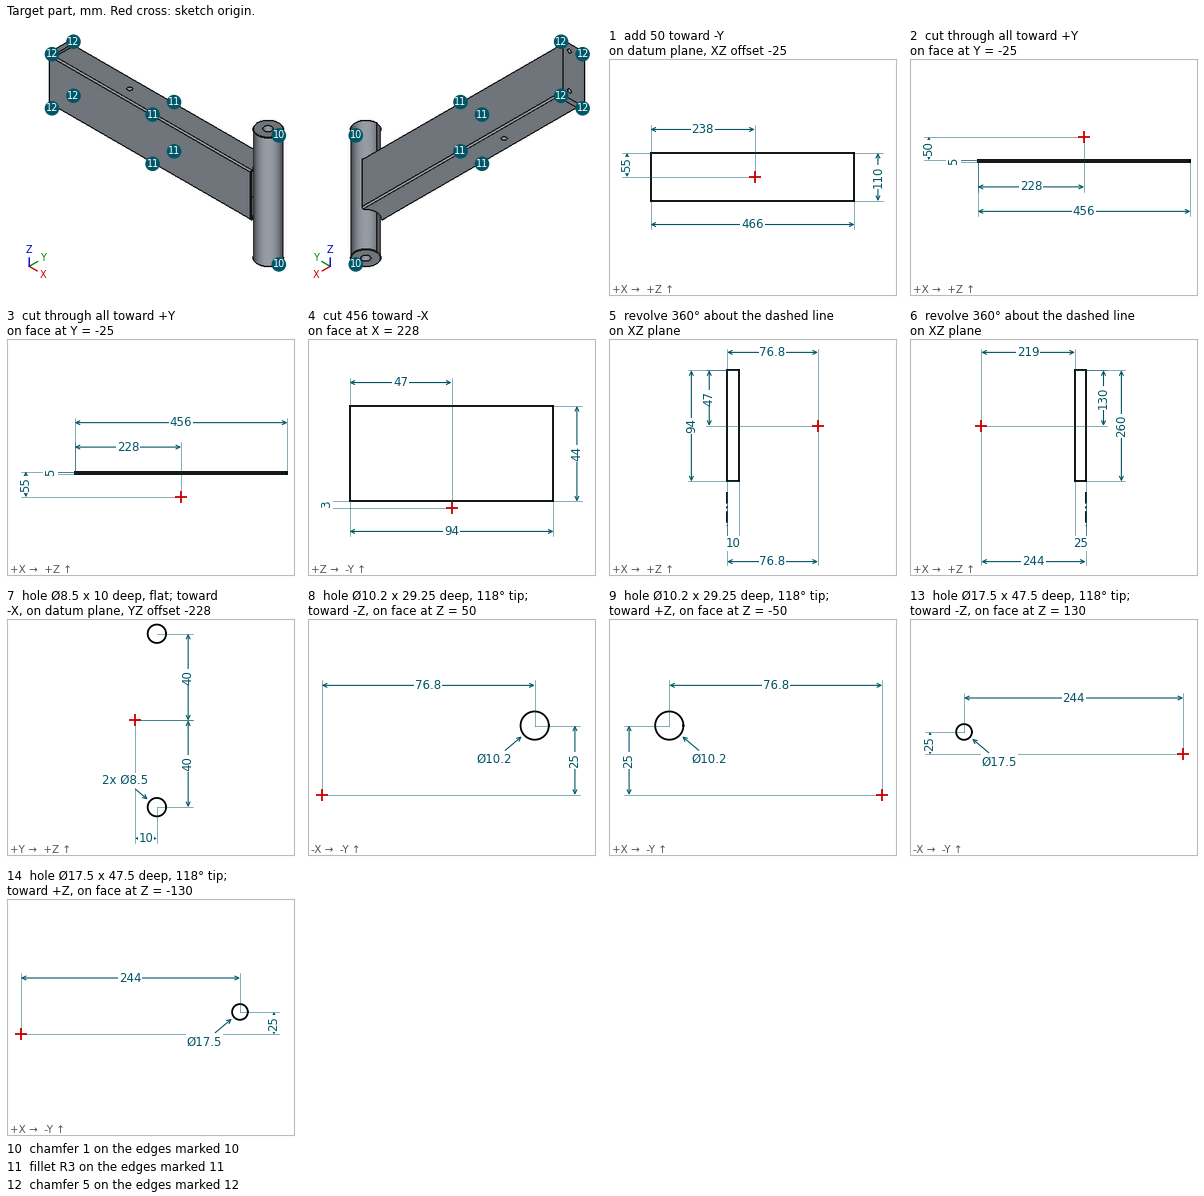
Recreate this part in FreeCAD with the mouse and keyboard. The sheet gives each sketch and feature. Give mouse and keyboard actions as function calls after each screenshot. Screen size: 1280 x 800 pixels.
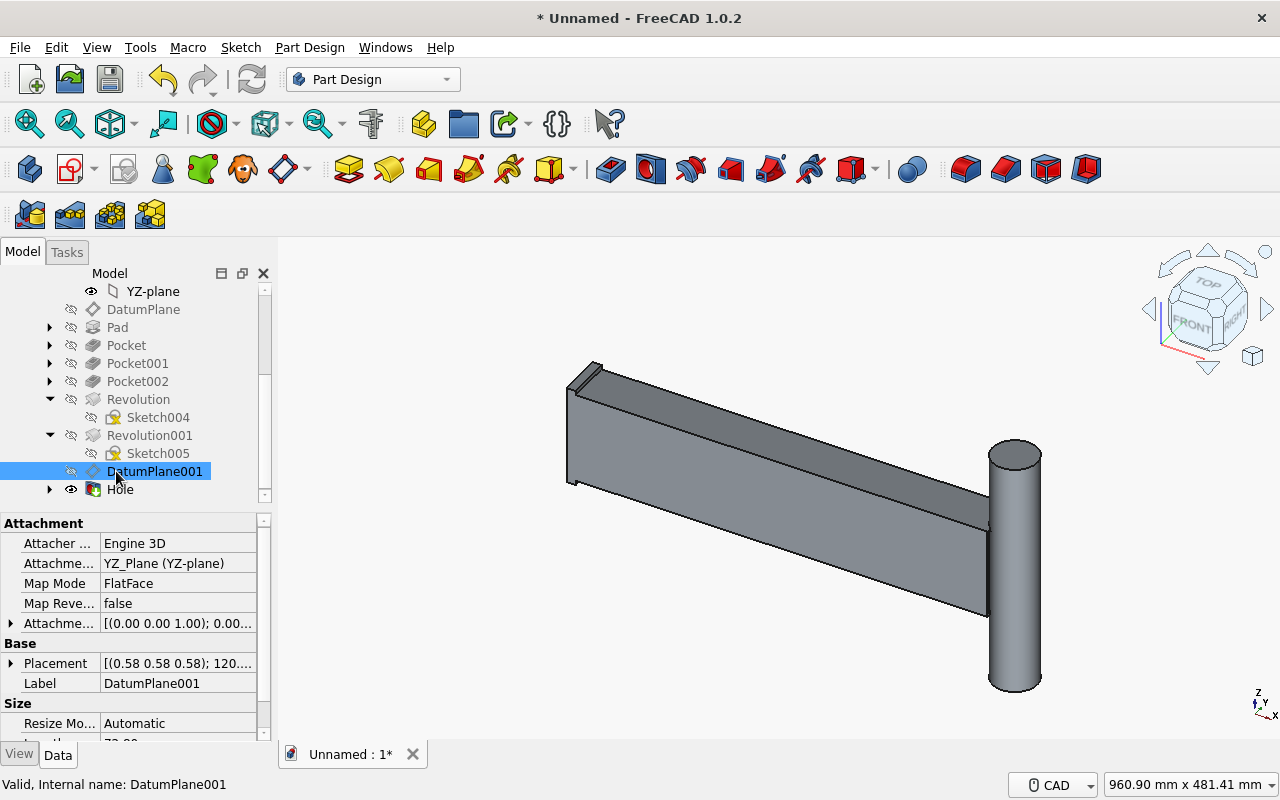
click(912, 488)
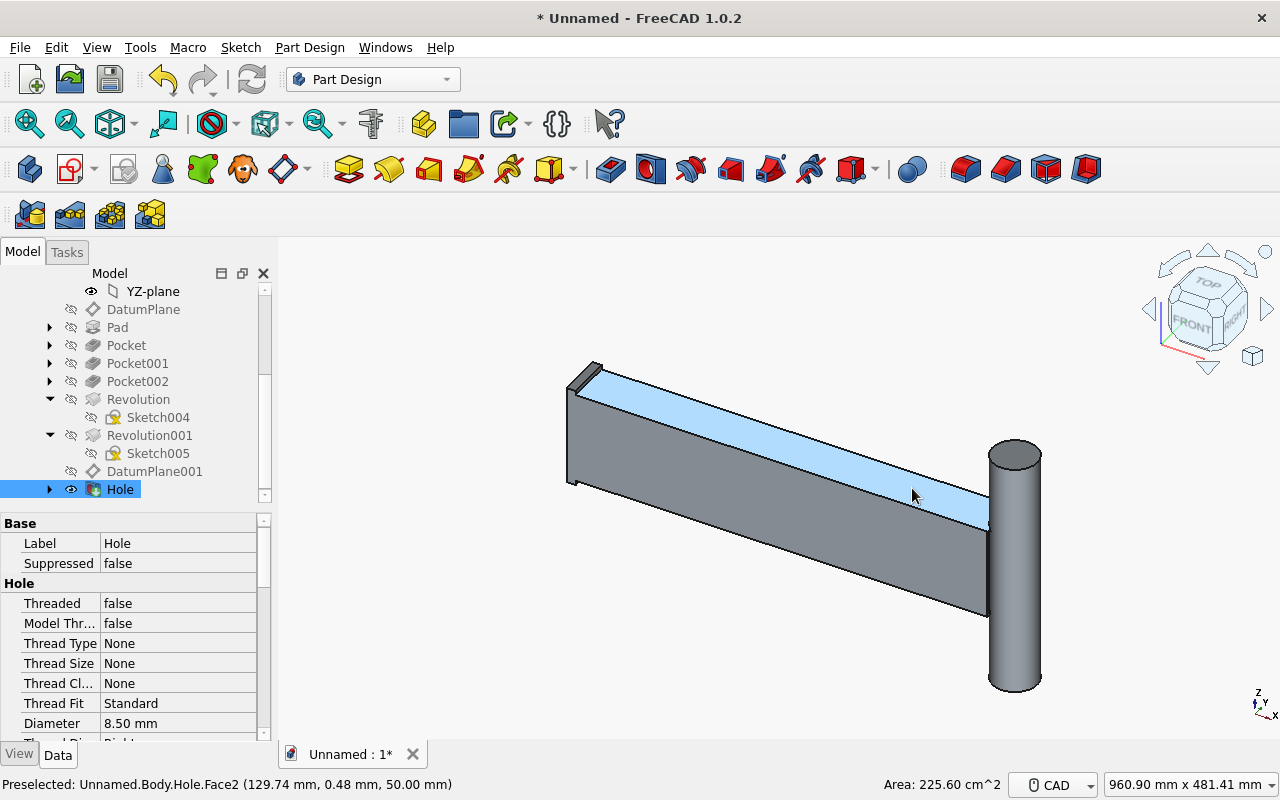
click(70, 170)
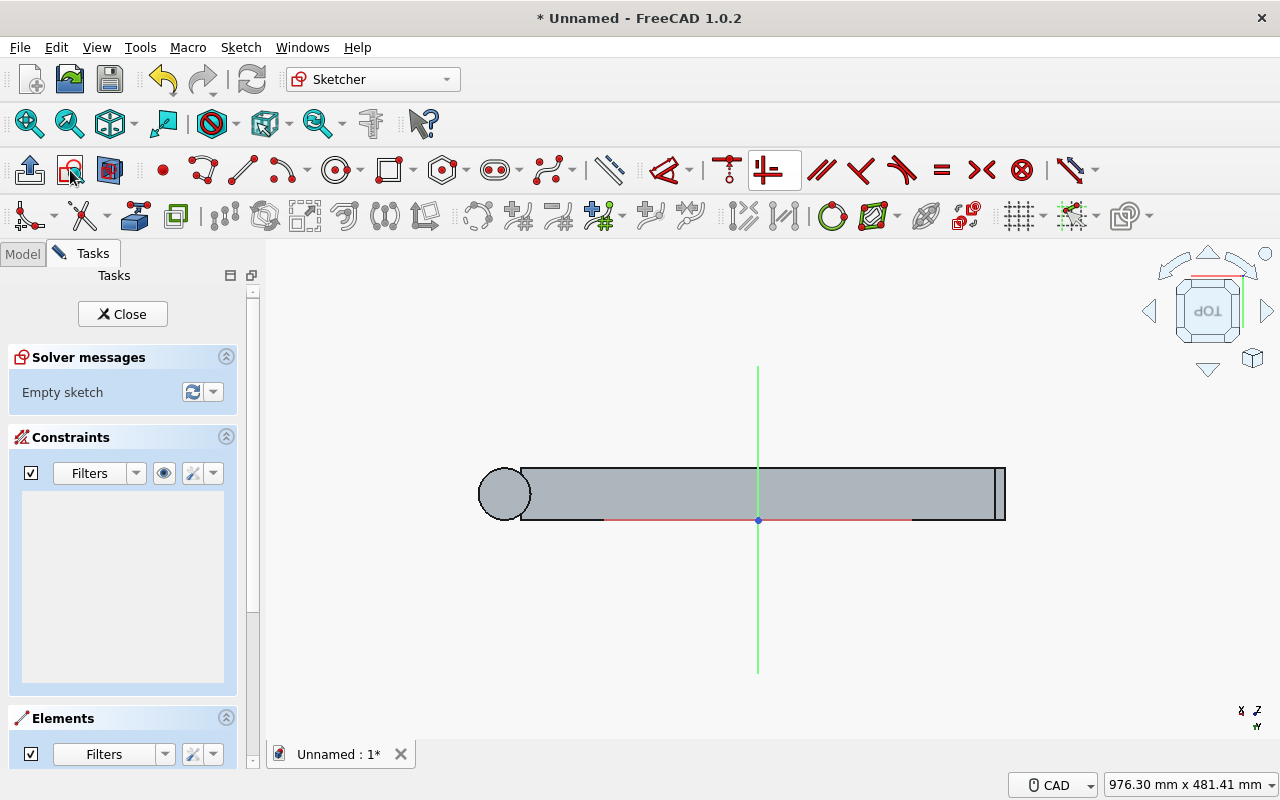
scroll(845, 494, up, 15)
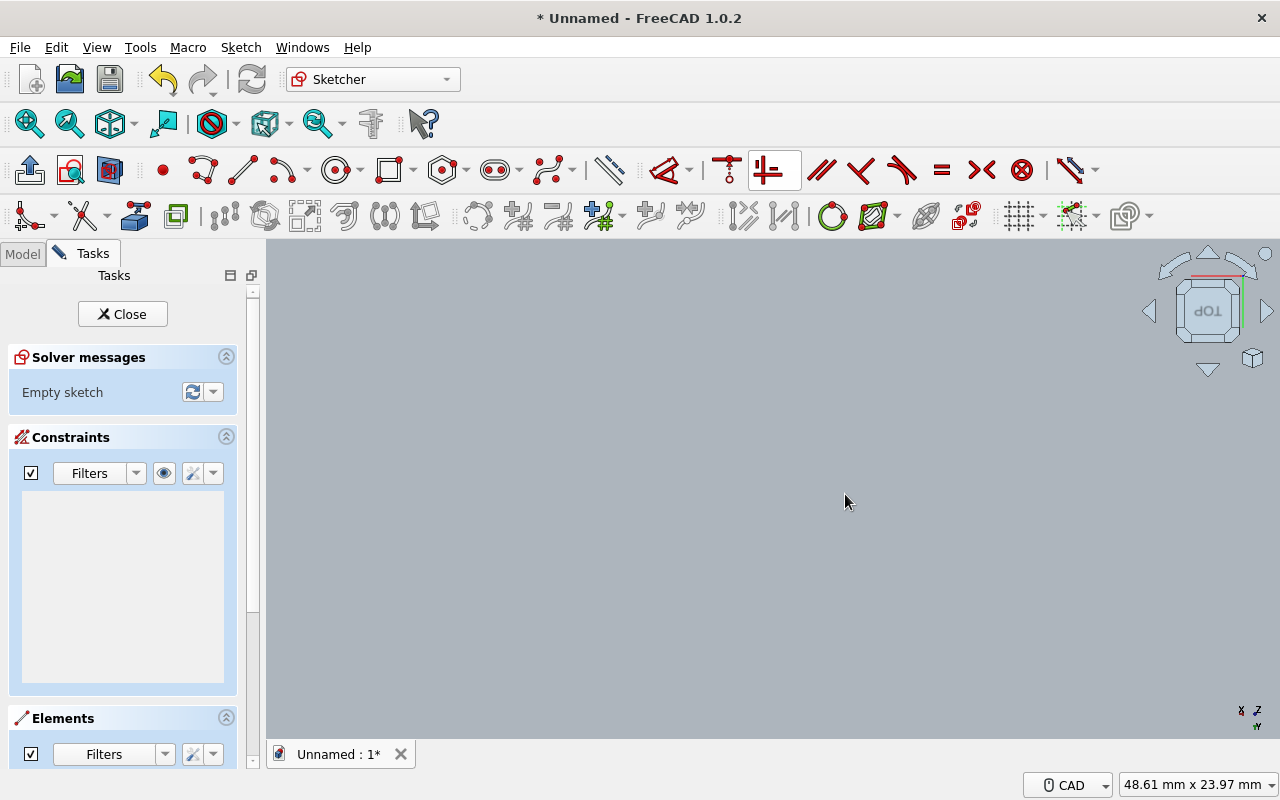
scroll(658, 481, up, 2)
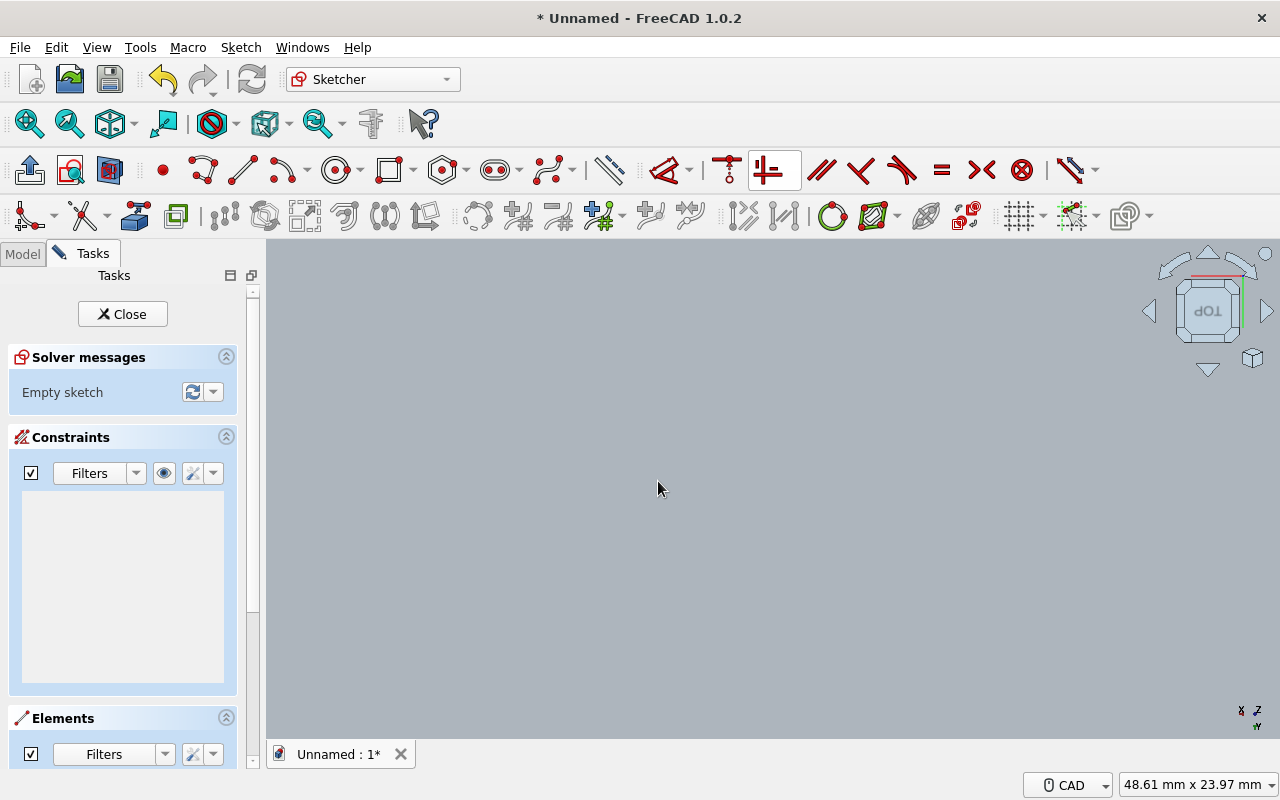
click(336, 170)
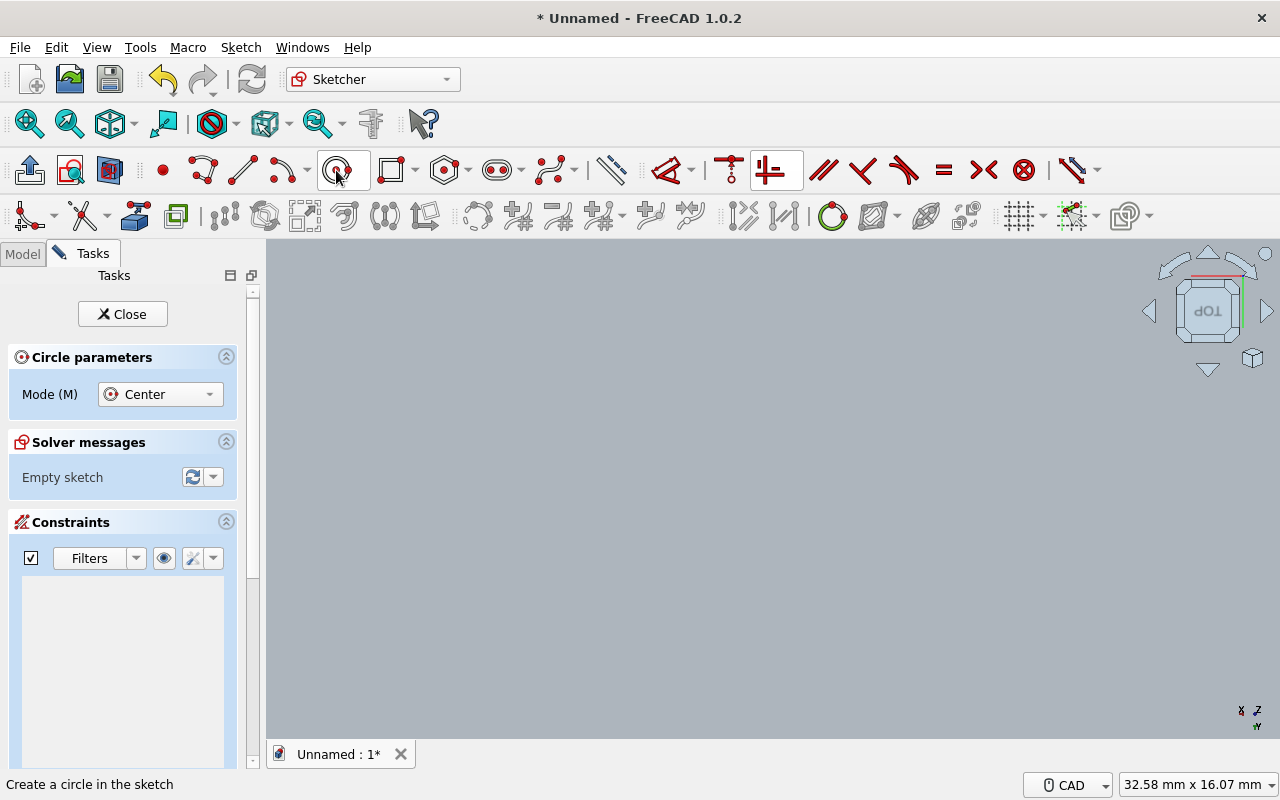
click(704, 489)
move(817, 376)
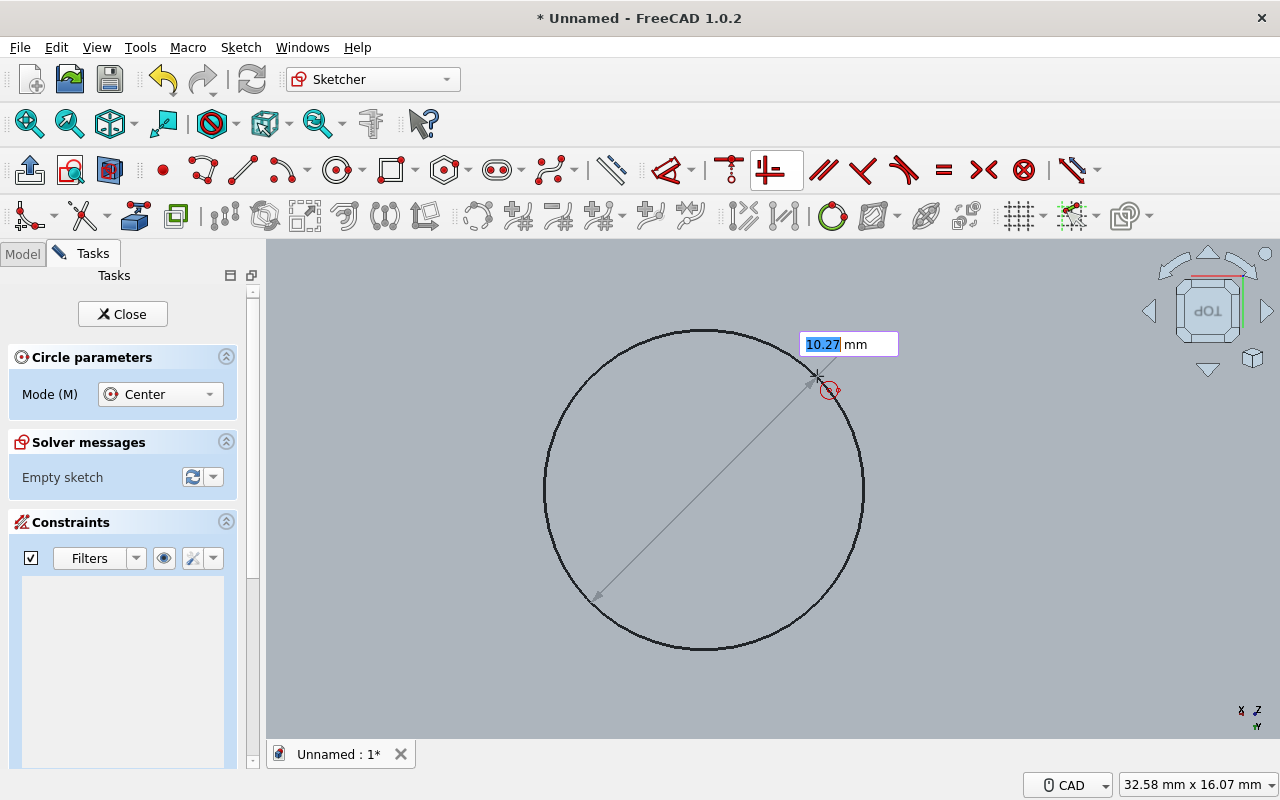
text(10.2)
key(Return)
key(Escape)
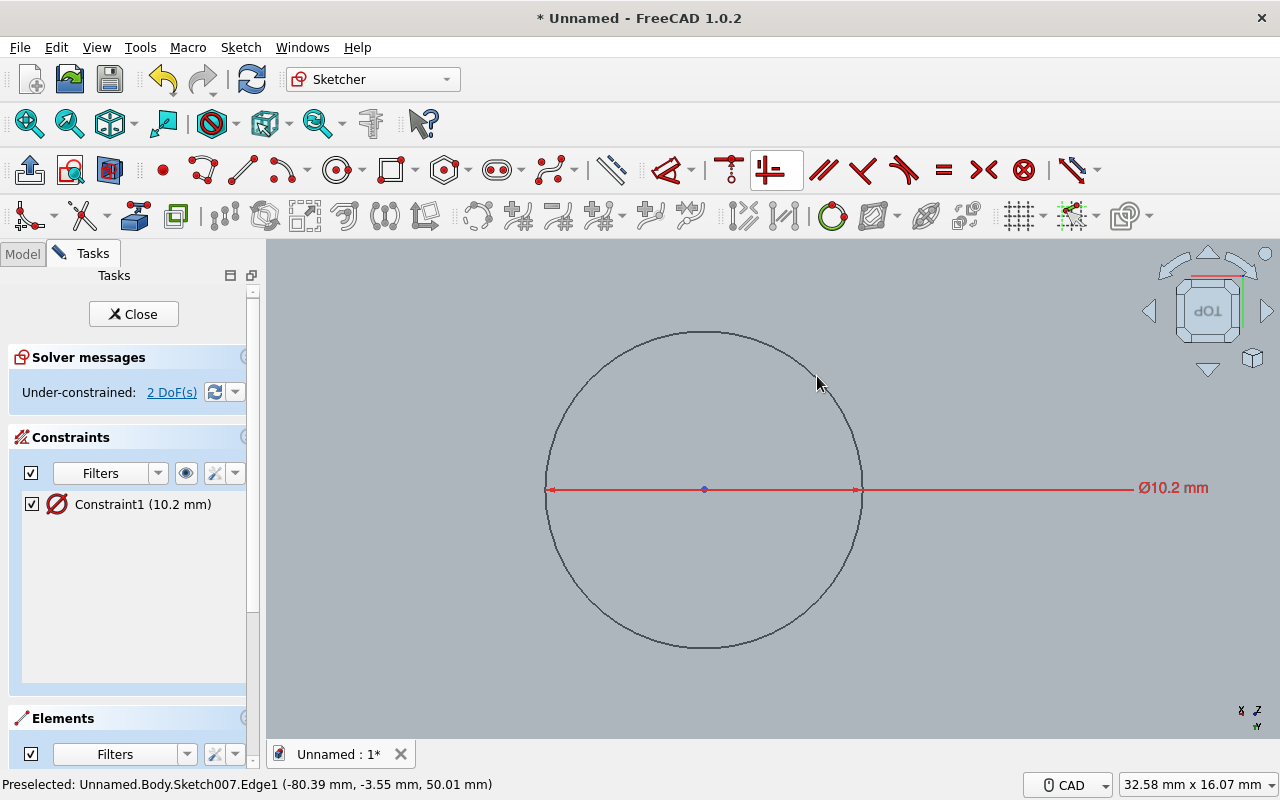
click(666, 170)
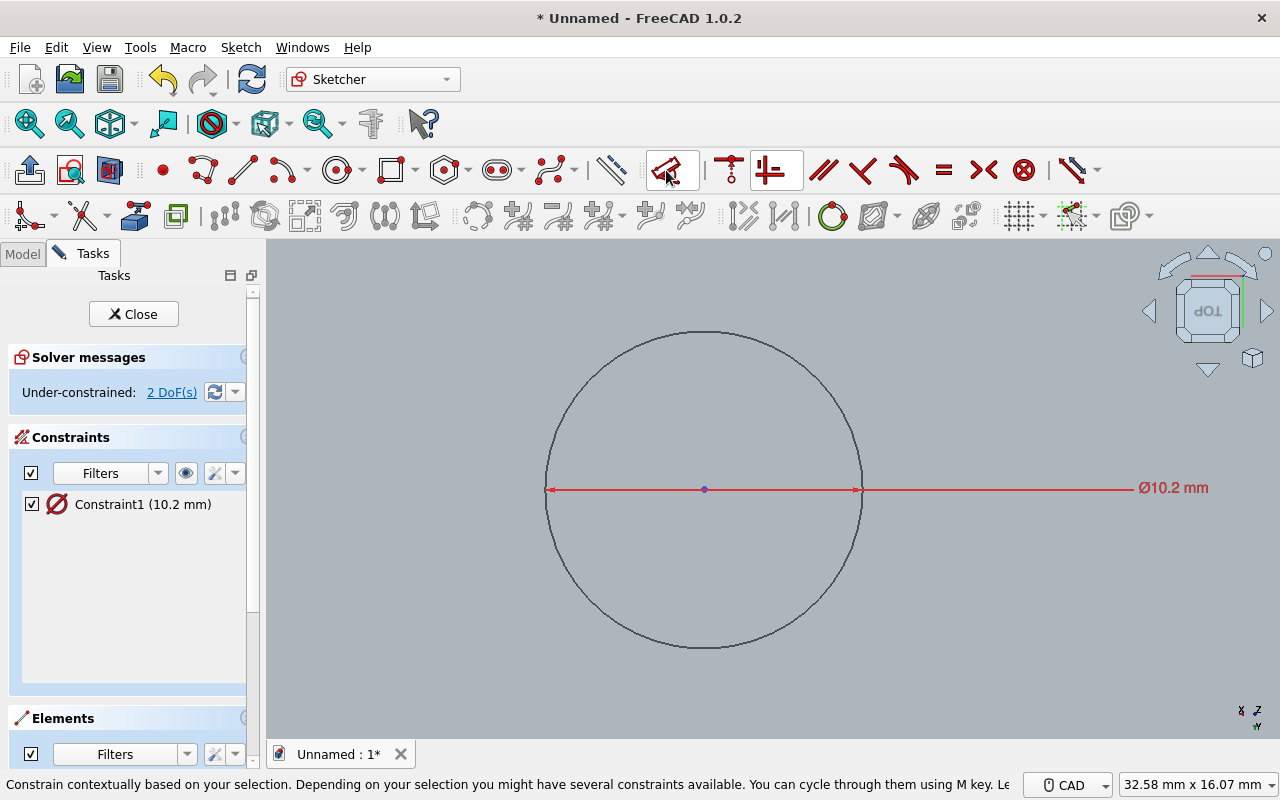
click(704, 490)
click(738, 601)